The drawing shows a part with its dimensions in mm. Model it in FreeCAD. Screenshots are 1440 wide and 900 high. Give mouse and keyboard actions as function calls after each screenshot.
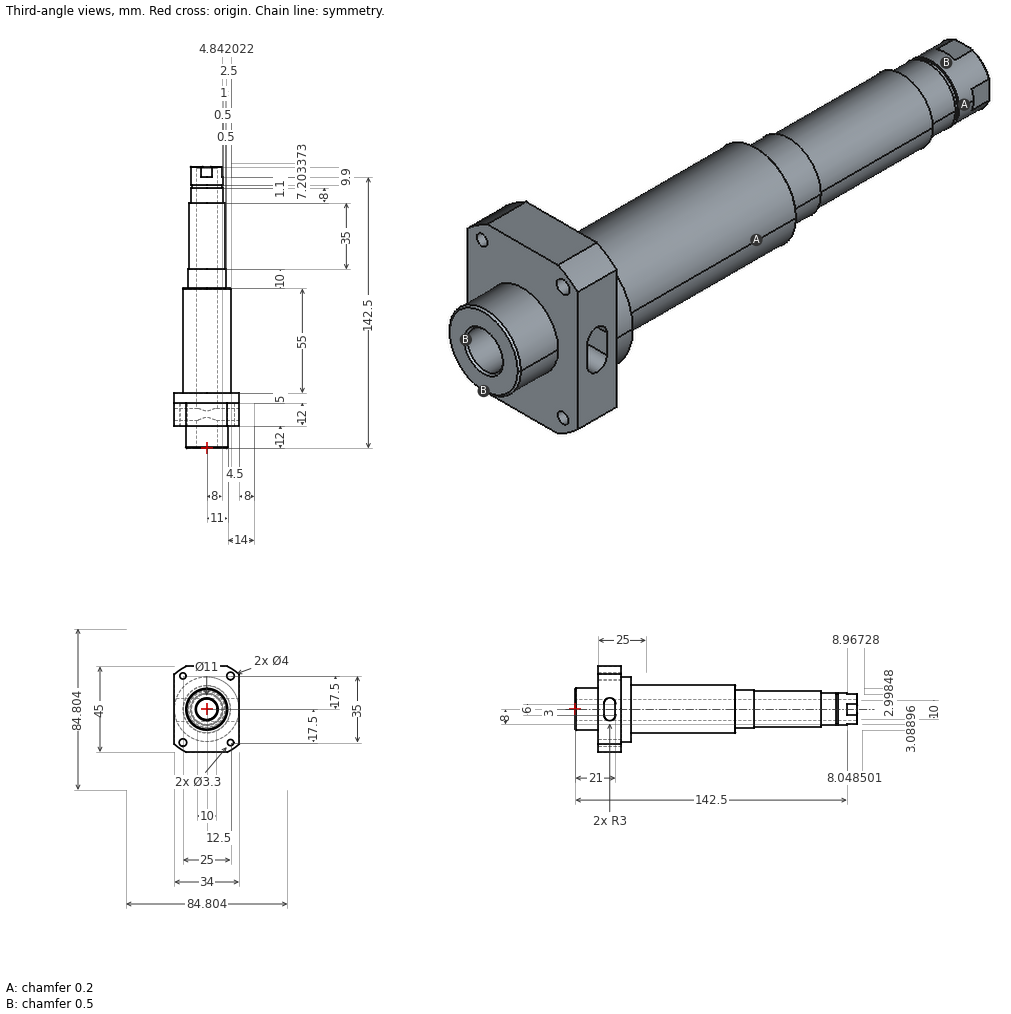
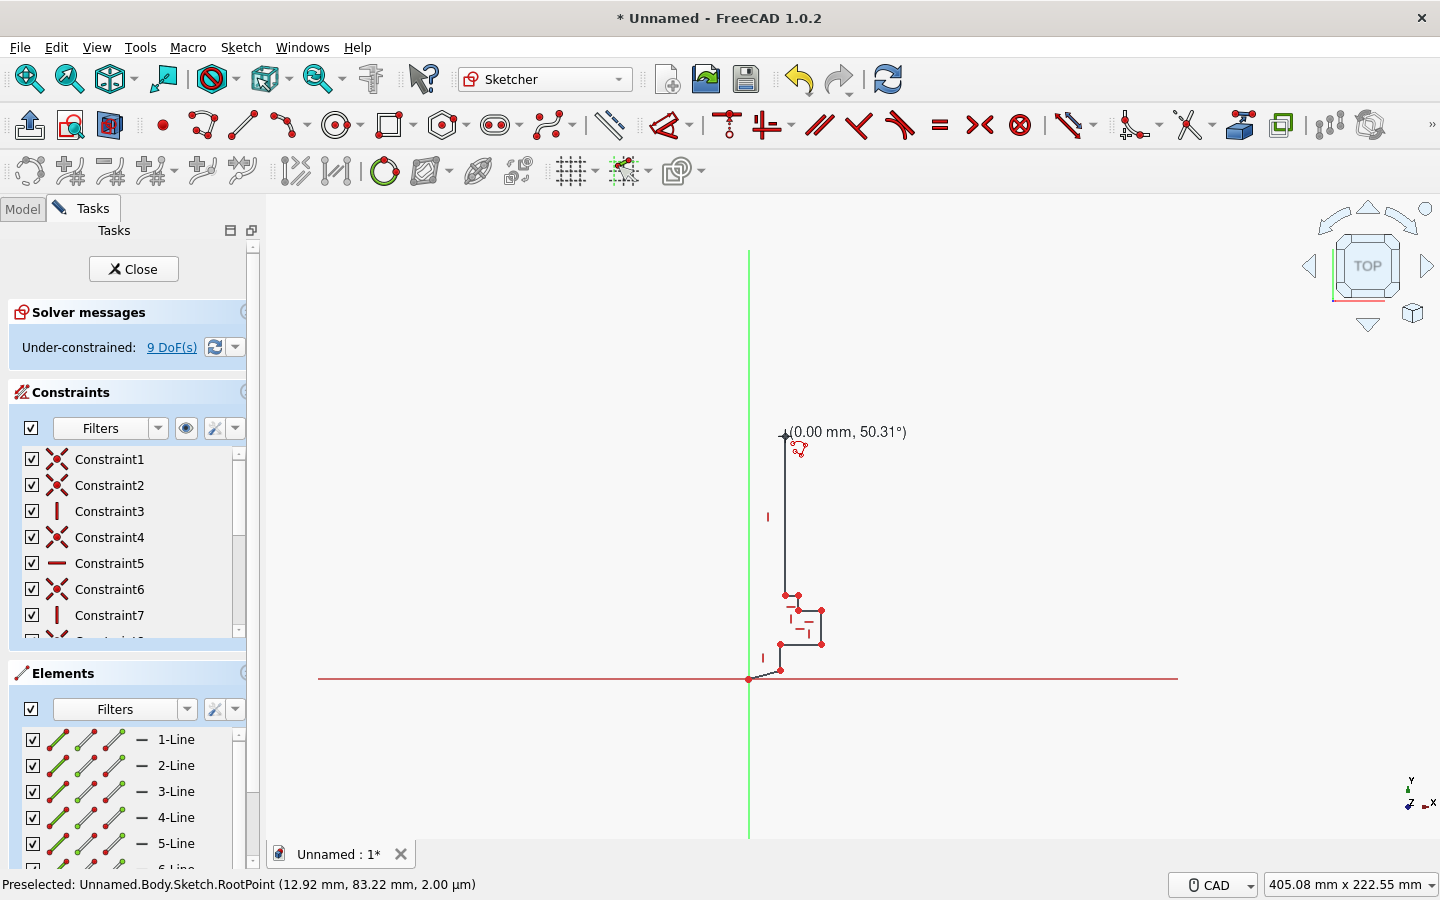
scroll(778, 436, up, 4)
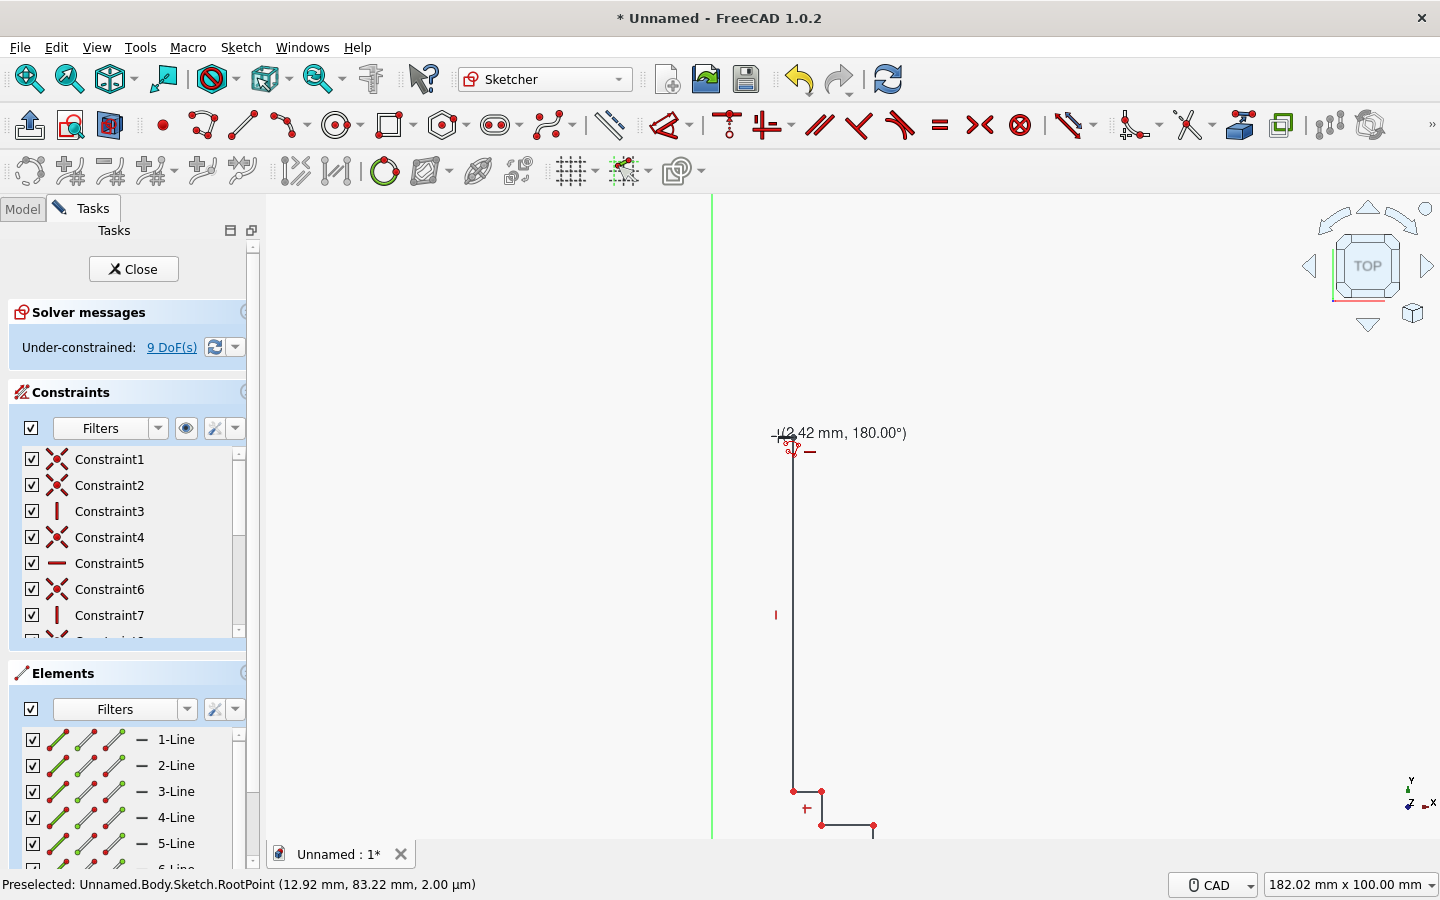
click(776, 436)
click(776, 370)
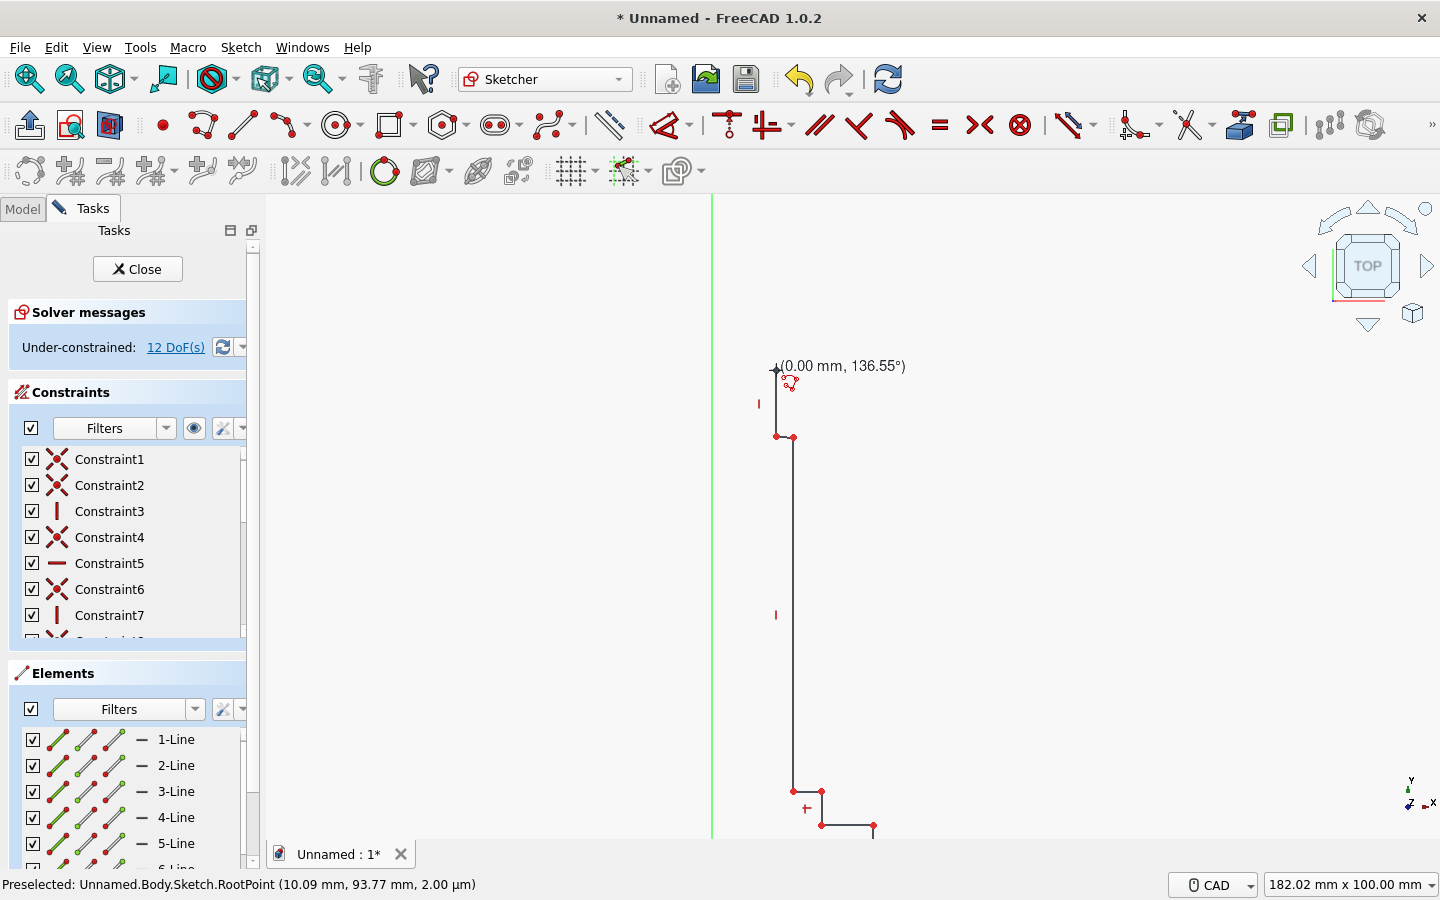
scroll(773, 370, up, 8)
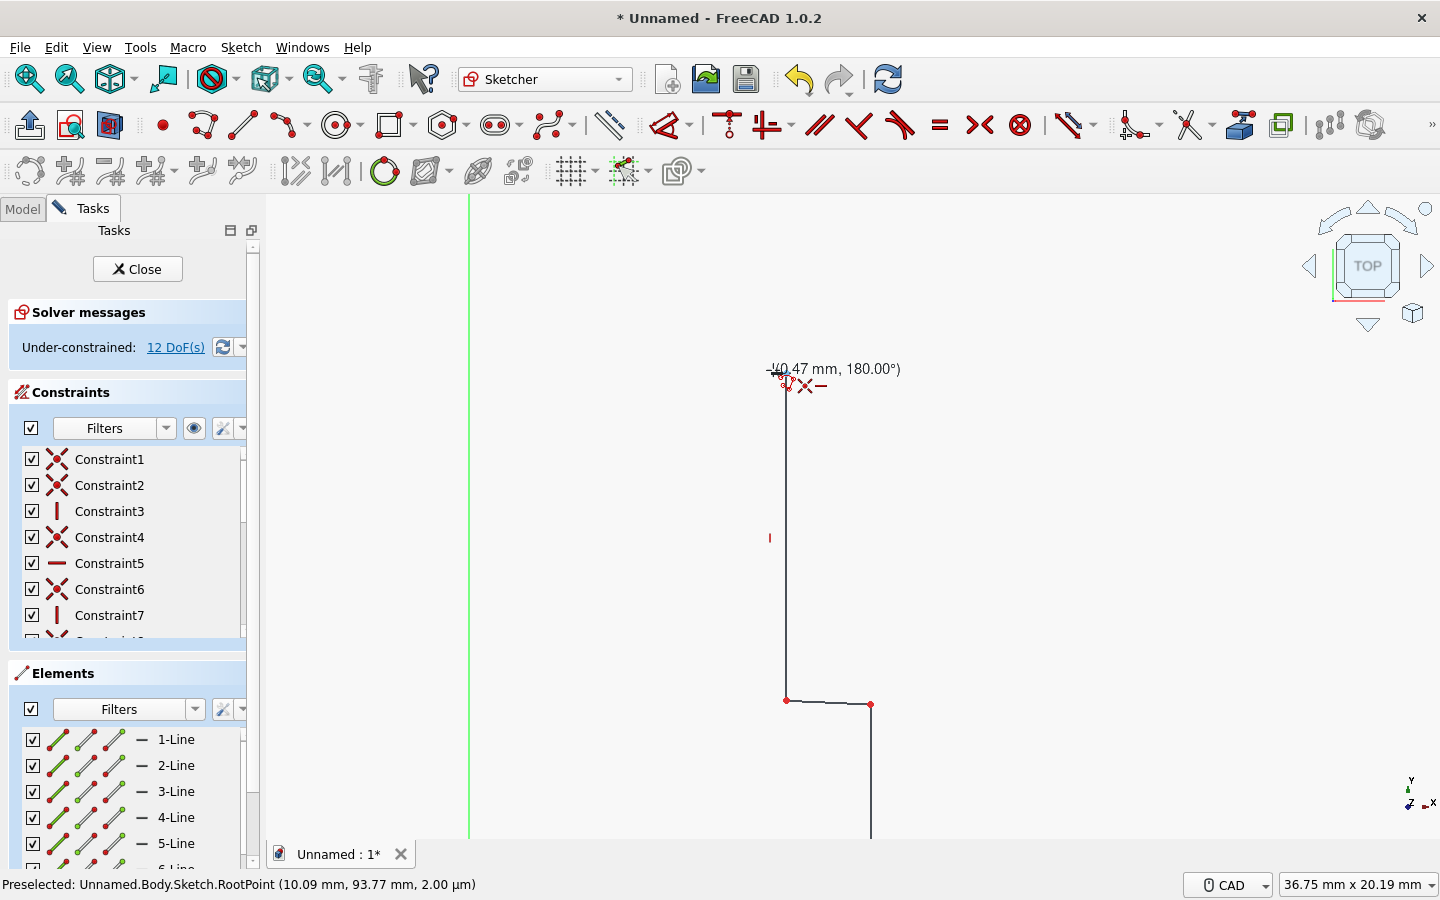
click(772, 369)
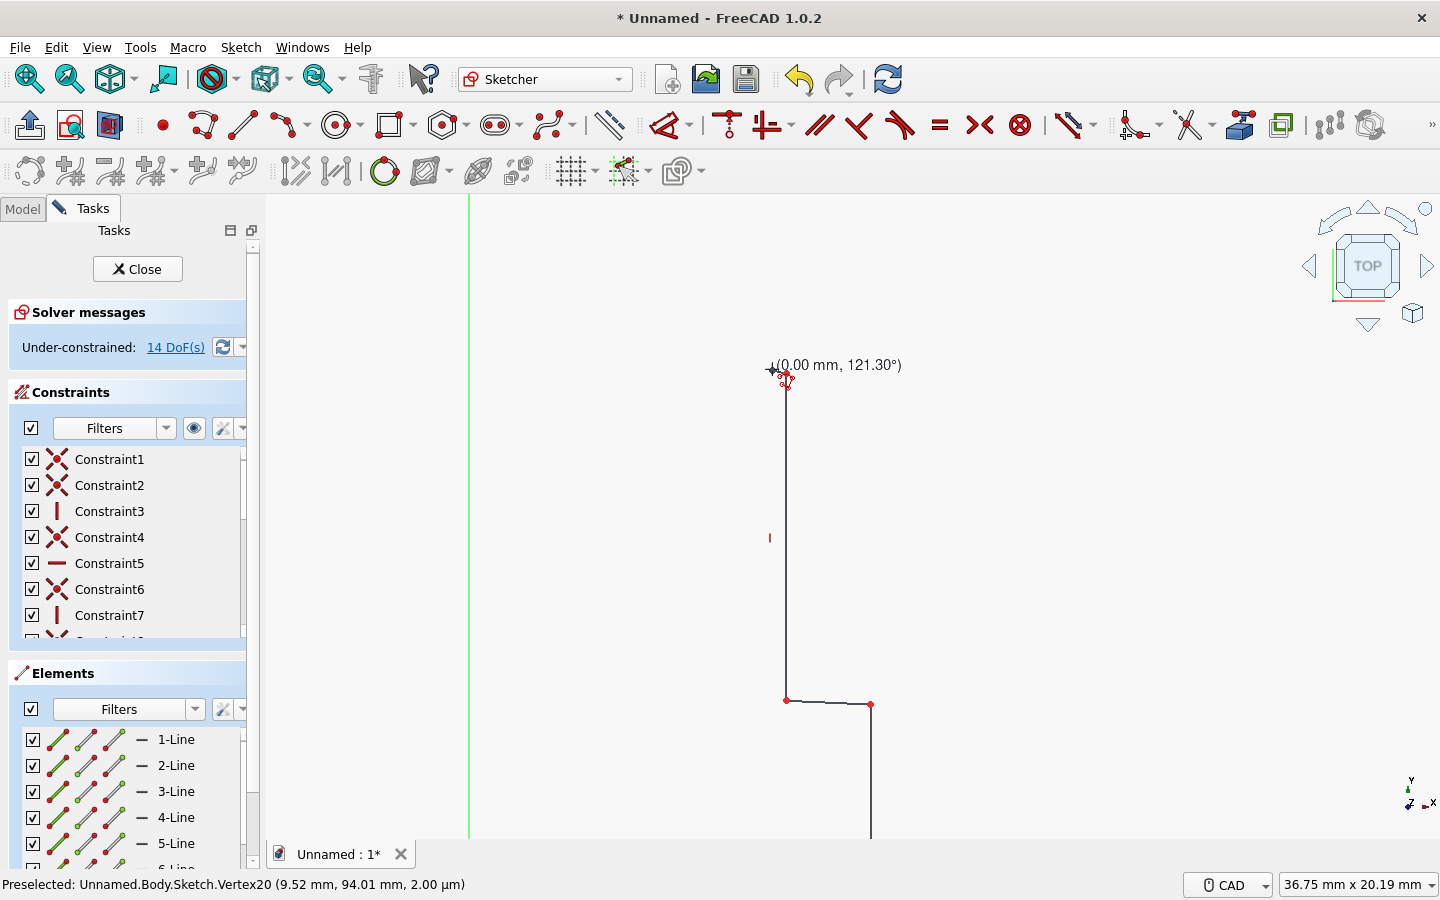
scroll(776, 467, down, 12)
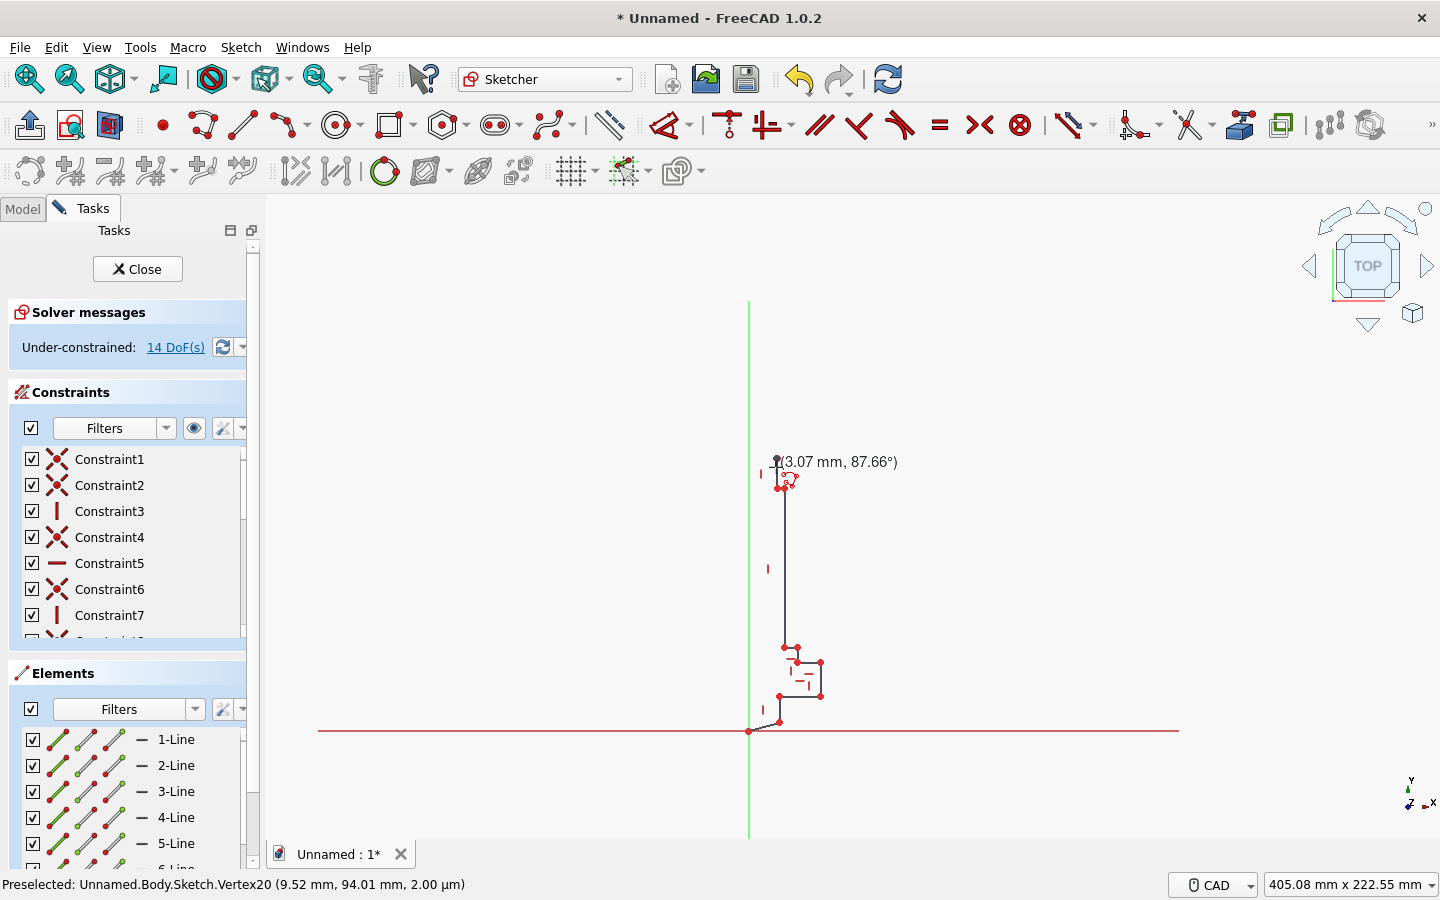
click(776, 357)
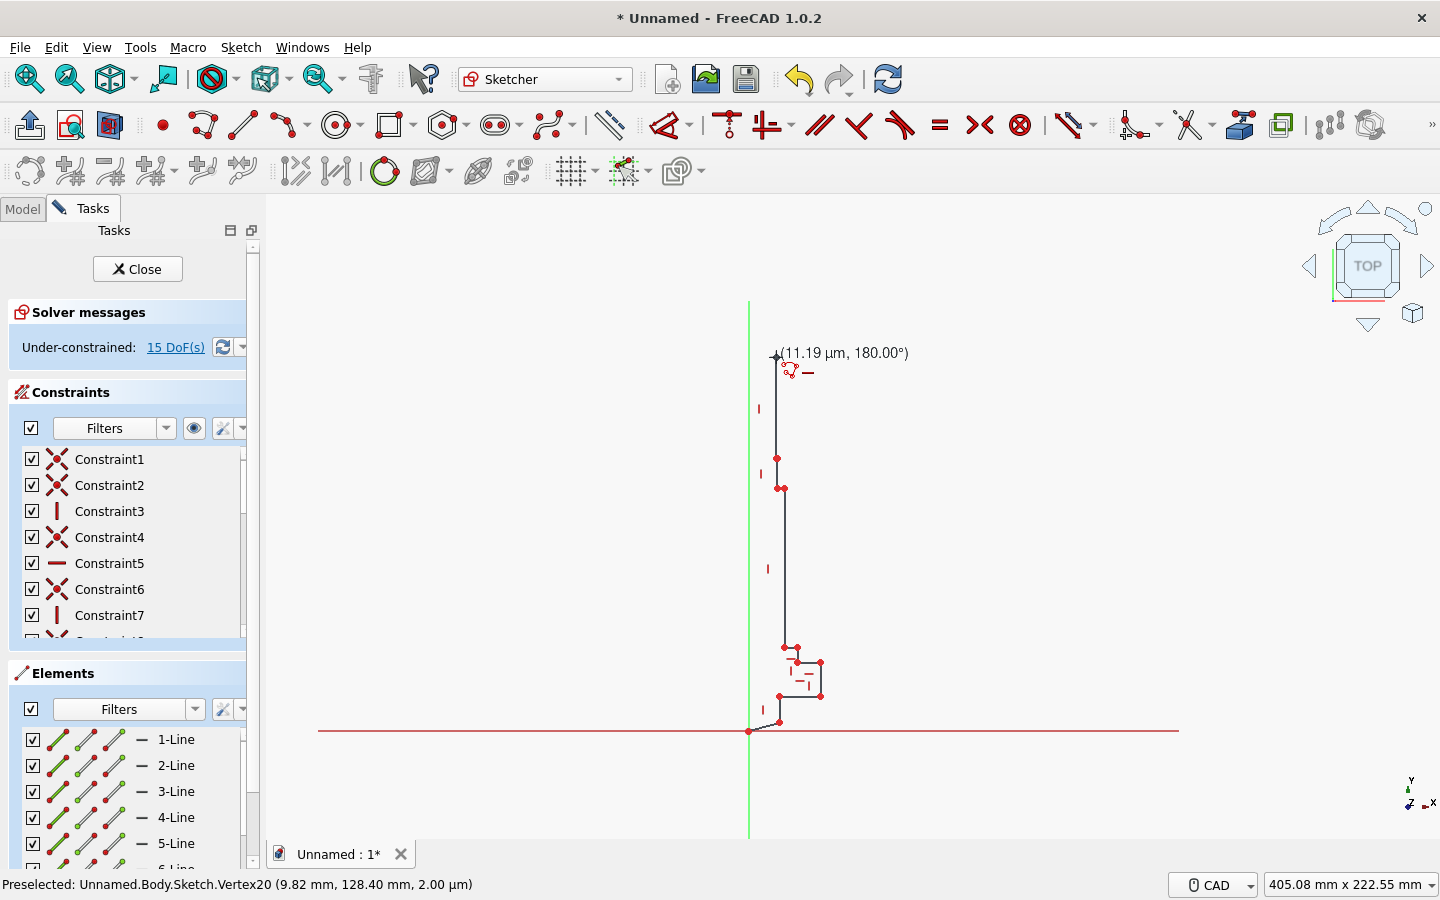
scroll(773, 357, up, 9)